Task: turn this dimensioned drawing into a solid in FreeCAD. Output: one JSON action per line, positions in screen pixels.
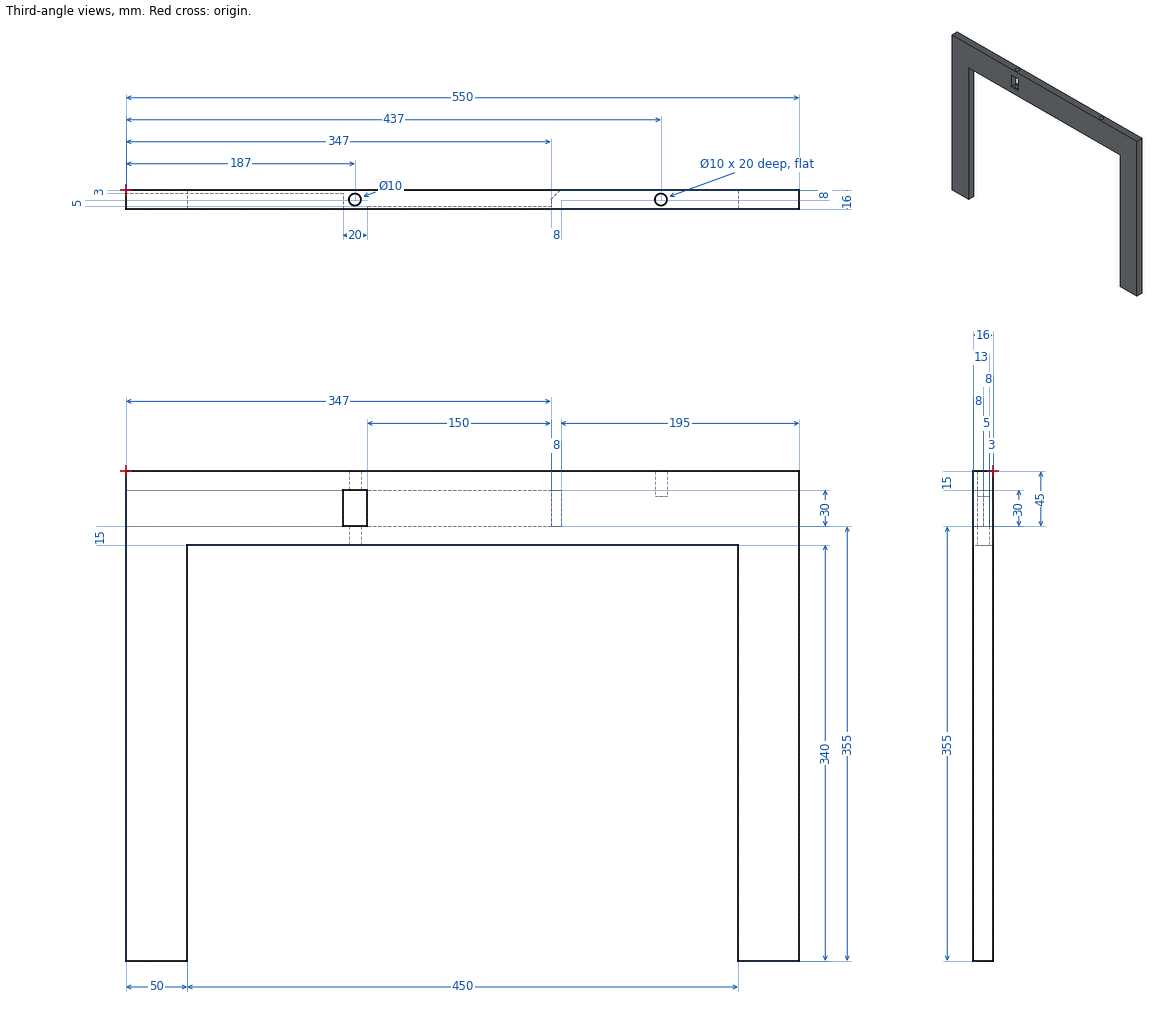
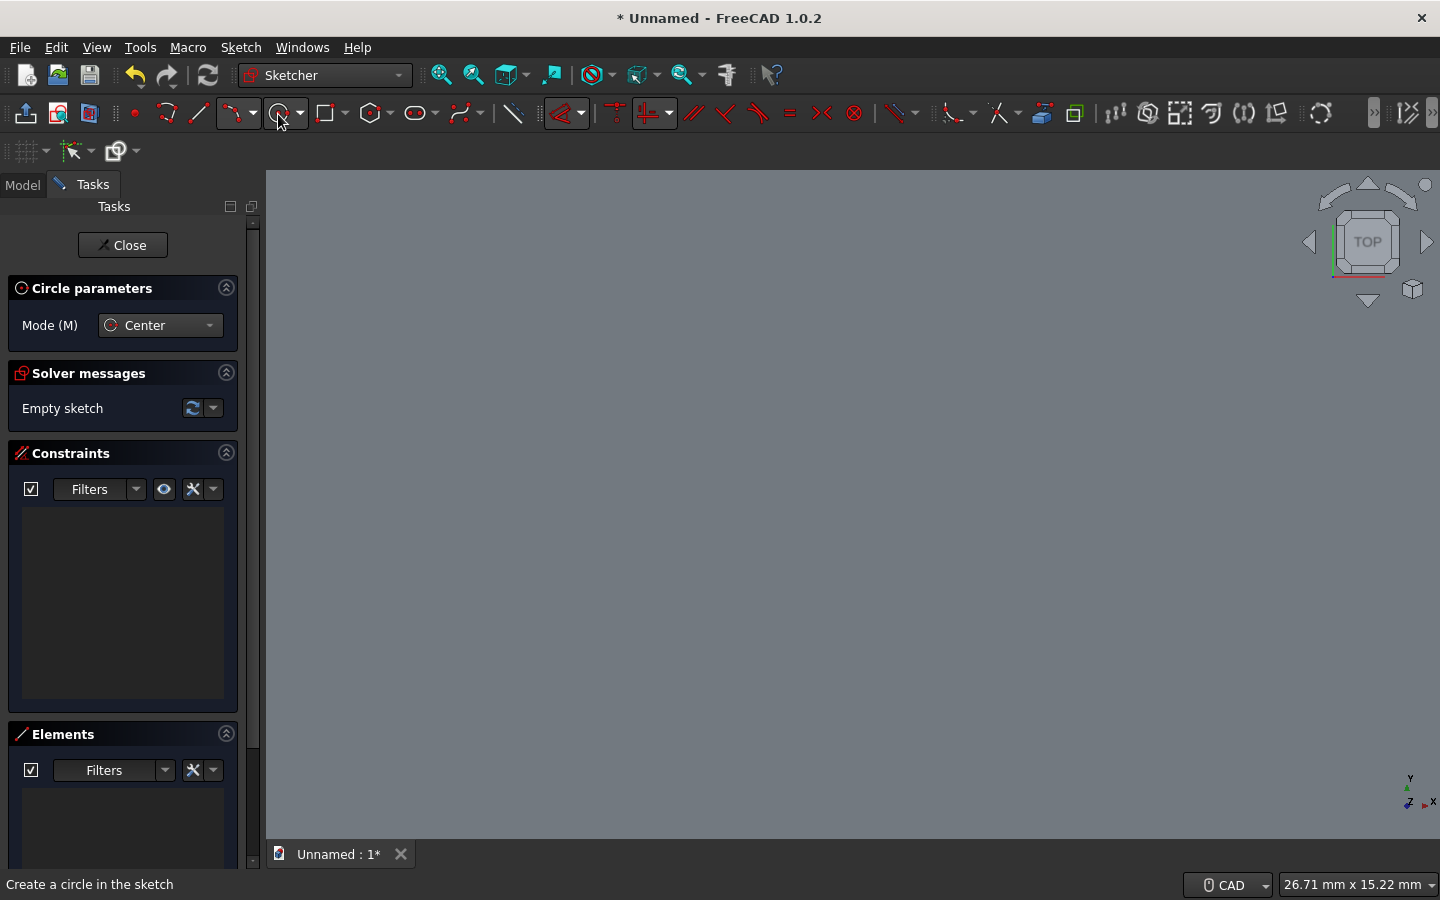
{"action": "left_click", "coordinate": [784, 504]}
{"action": "left_click", "coordinate": [939, 349]}
{"action": "key", "text": "Escape"}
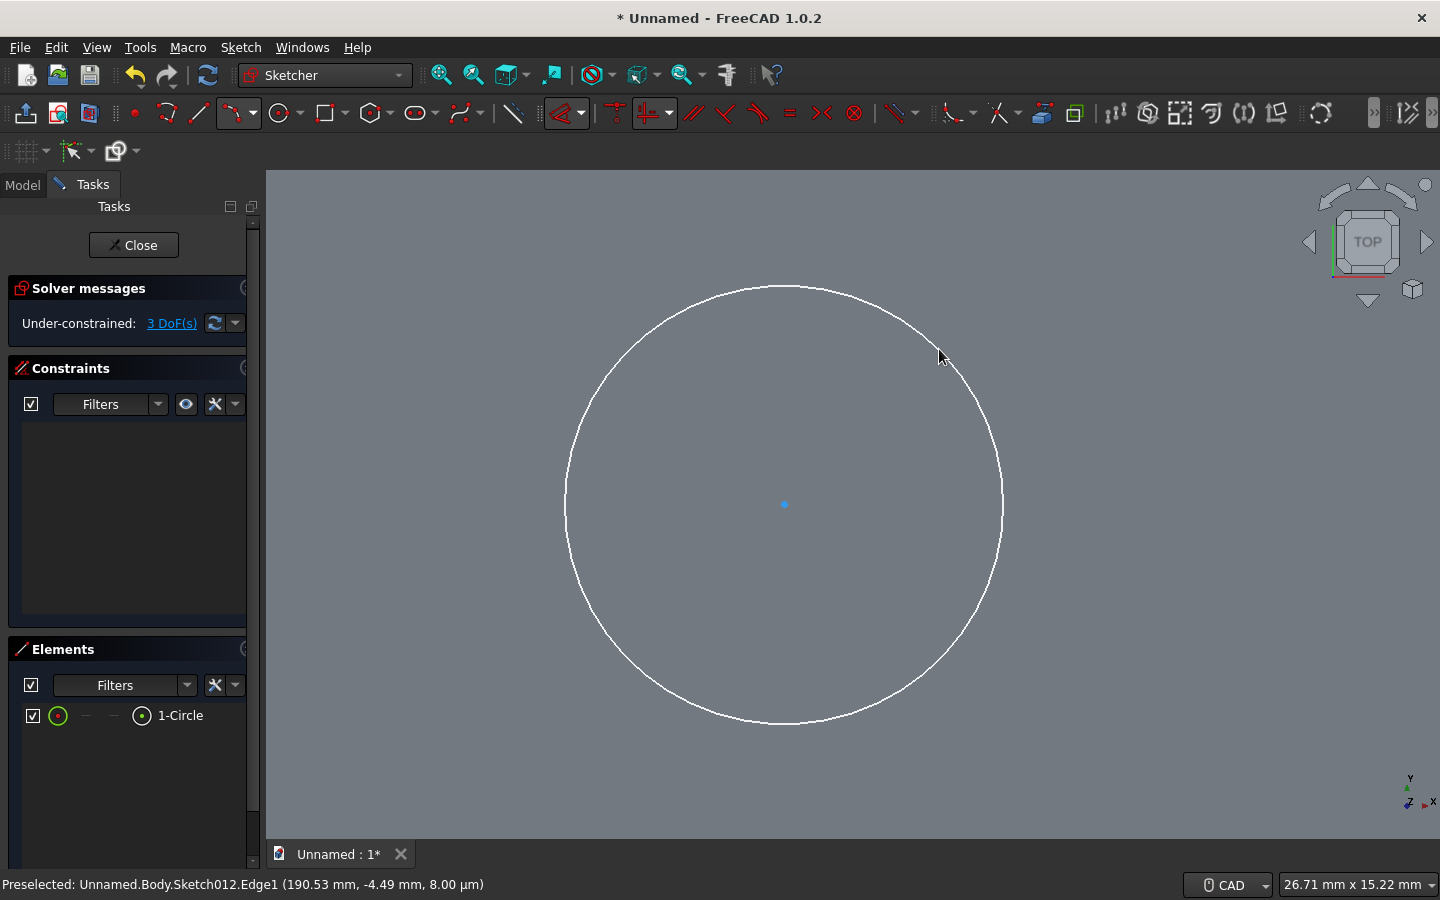
{"action": "left_click", "coordinate": [939, 350]}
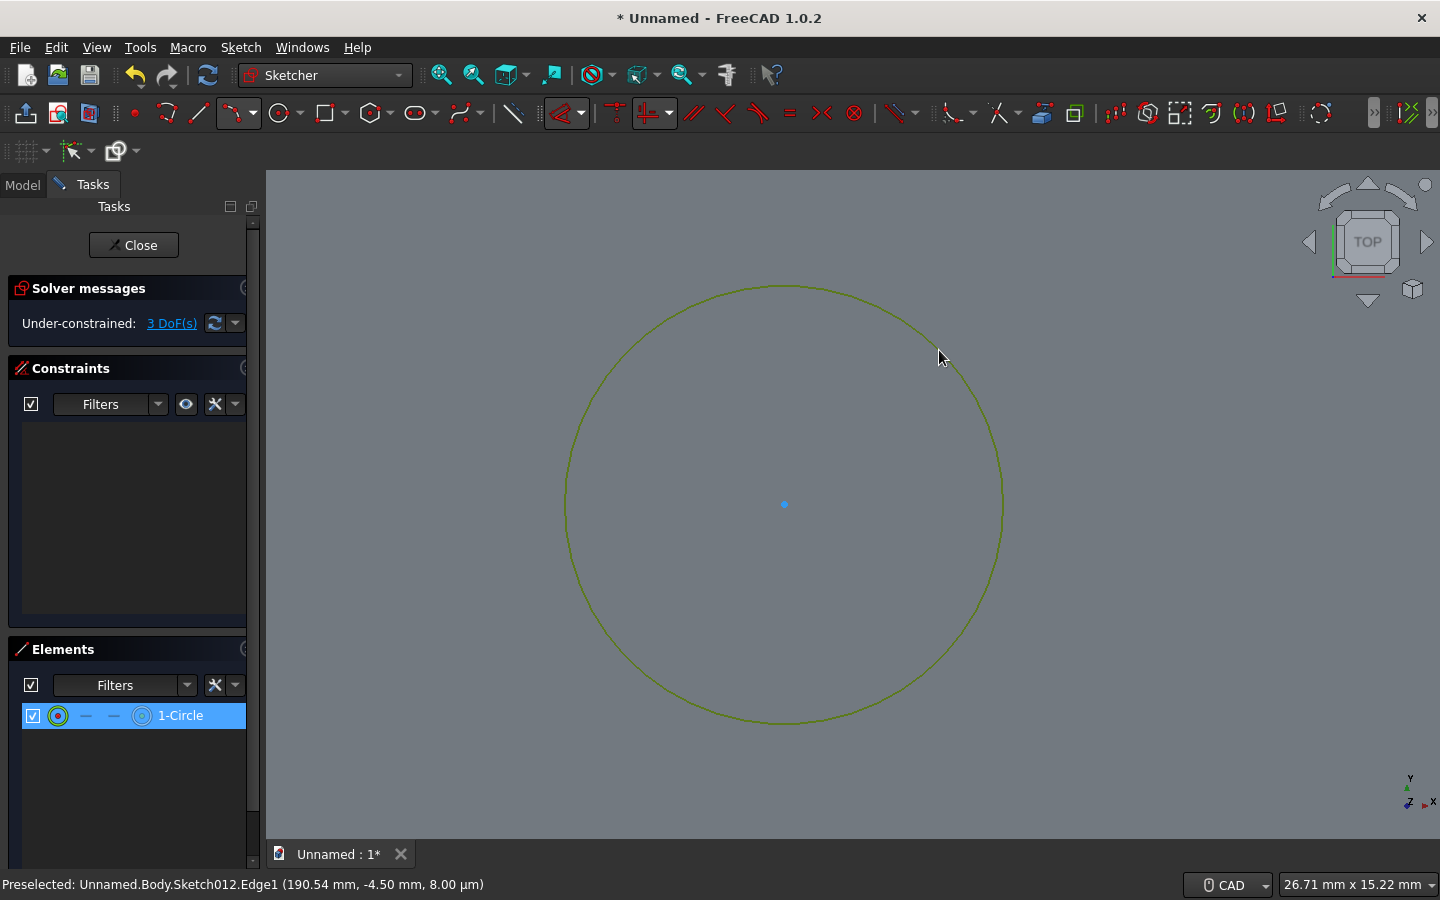
{"action": "key", "text": "k o"}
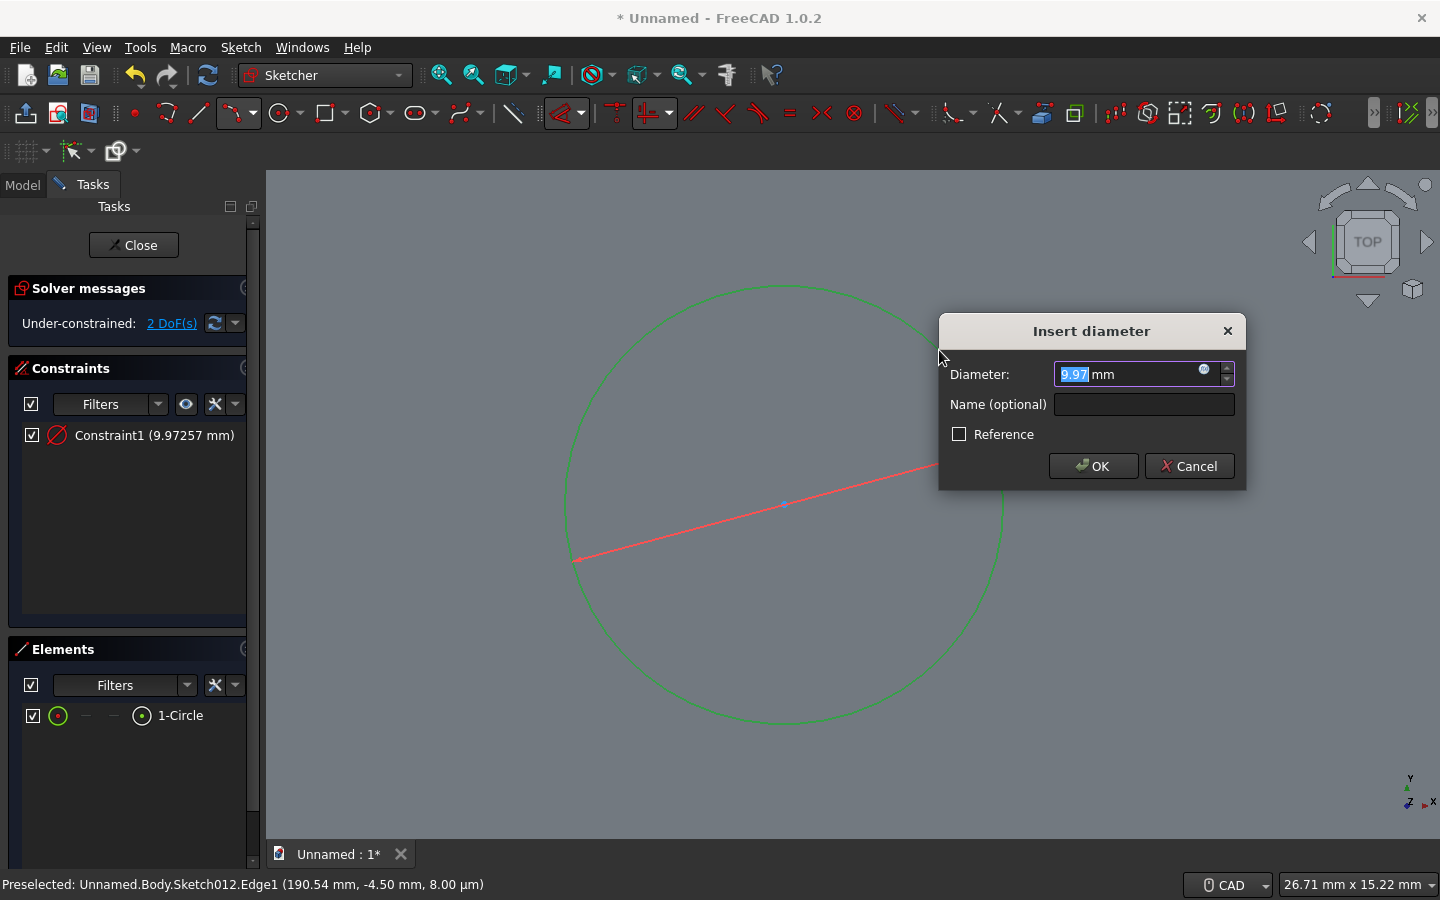
{"action": "type", "text": "10"}
{"action": "key", "text": "Return"}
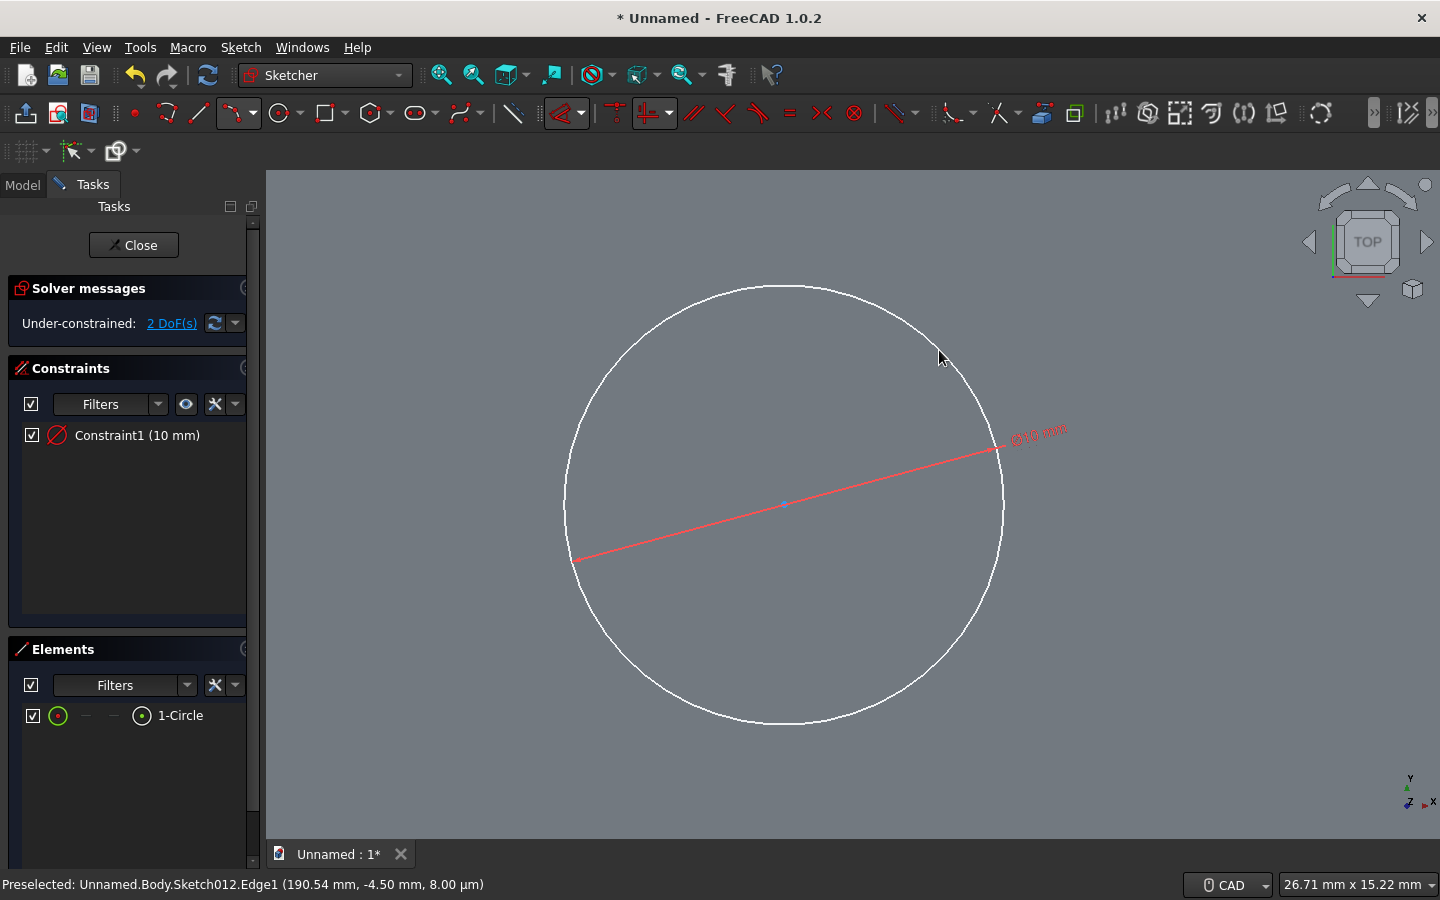
{"action": "left_click", "coordinate": [784, 505]}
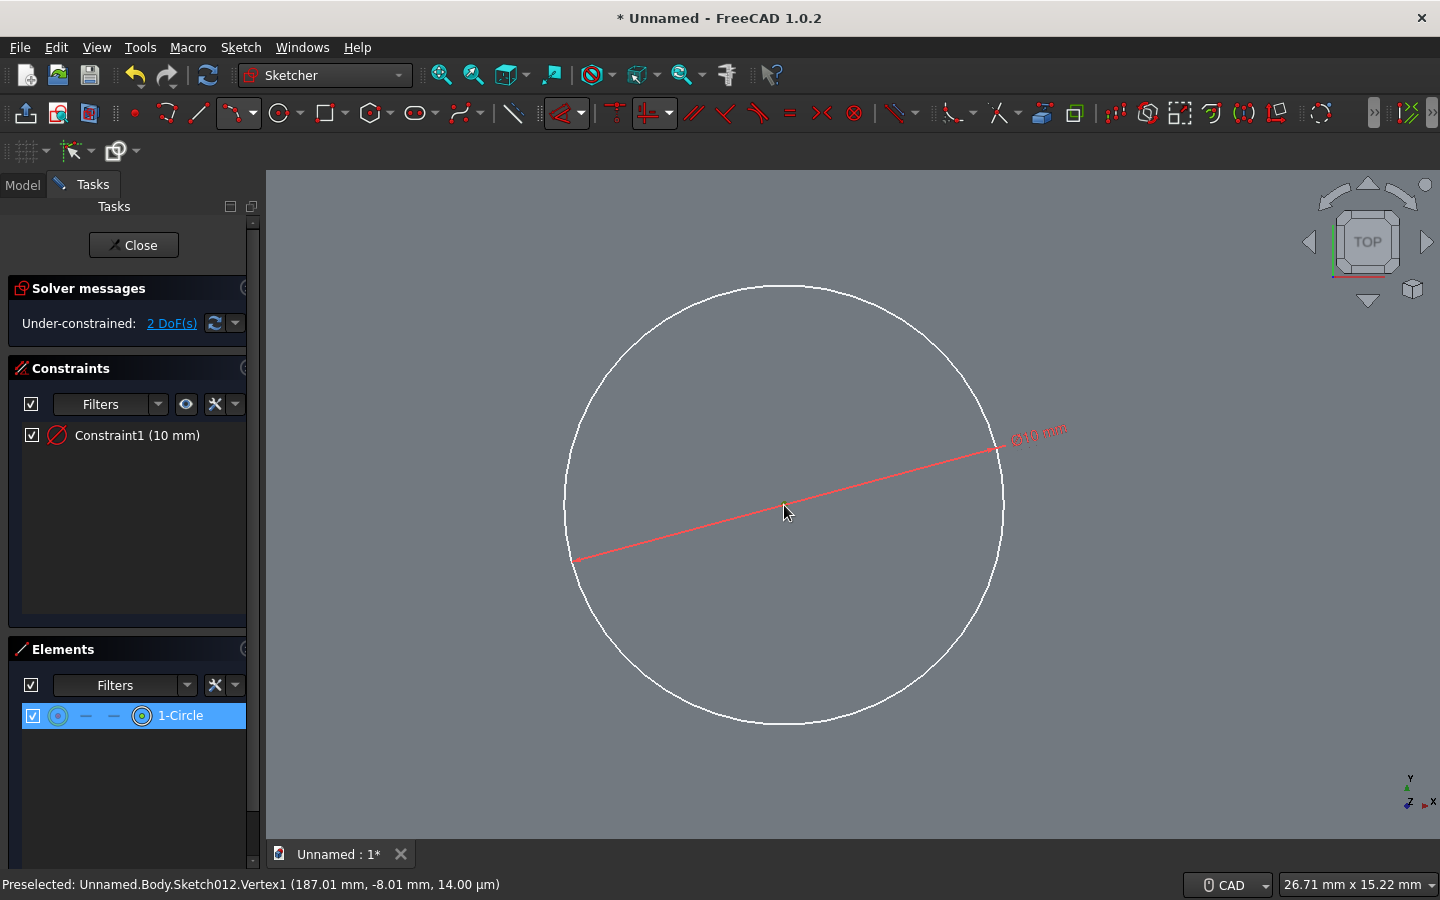
{"action": "key", "text": "i"}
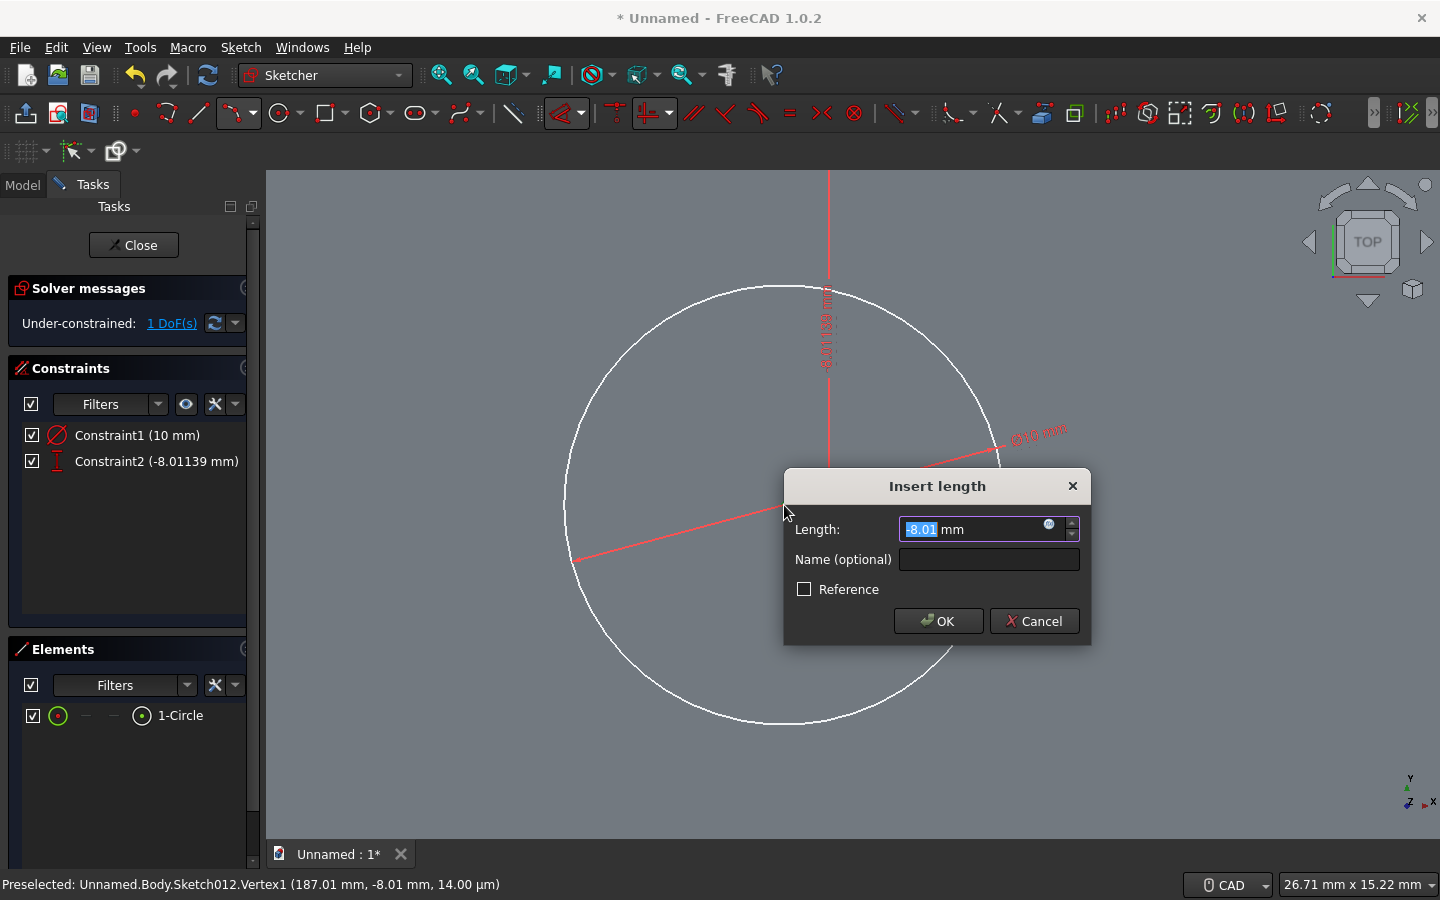
{"action": "type", "text": "-8"}
{"action": "key", "text": "Return"}